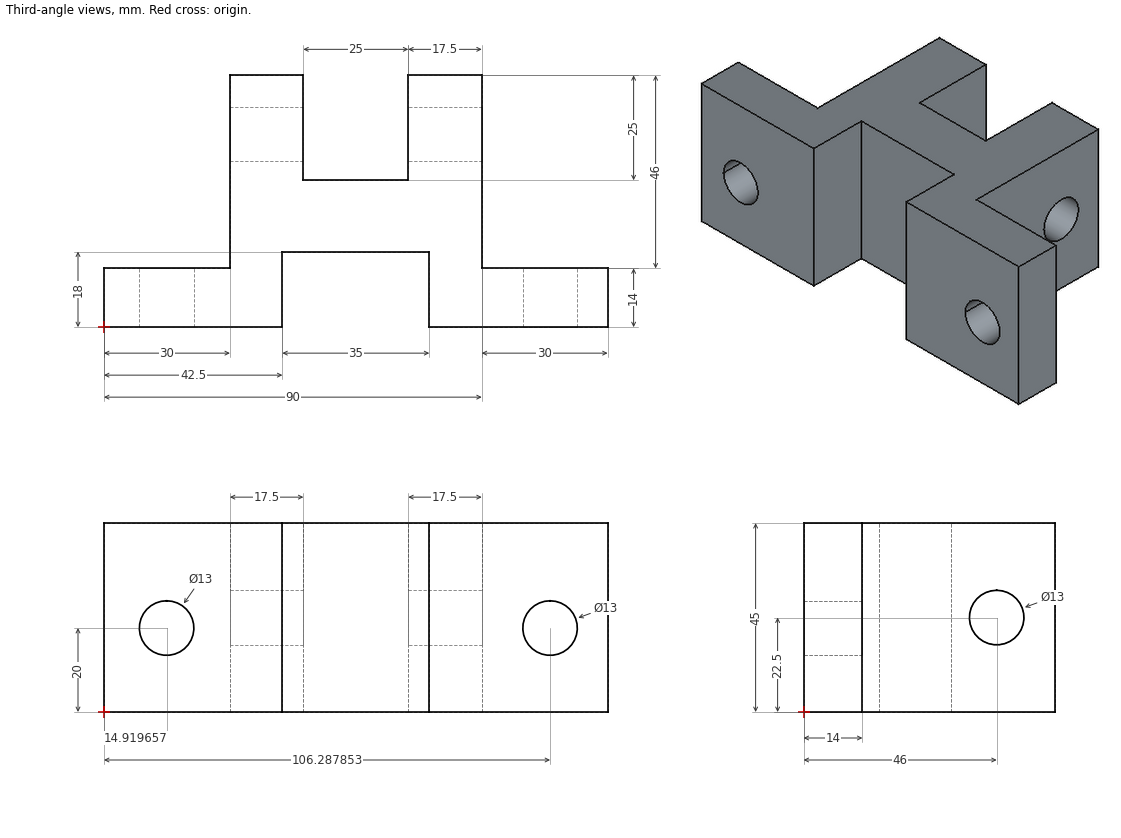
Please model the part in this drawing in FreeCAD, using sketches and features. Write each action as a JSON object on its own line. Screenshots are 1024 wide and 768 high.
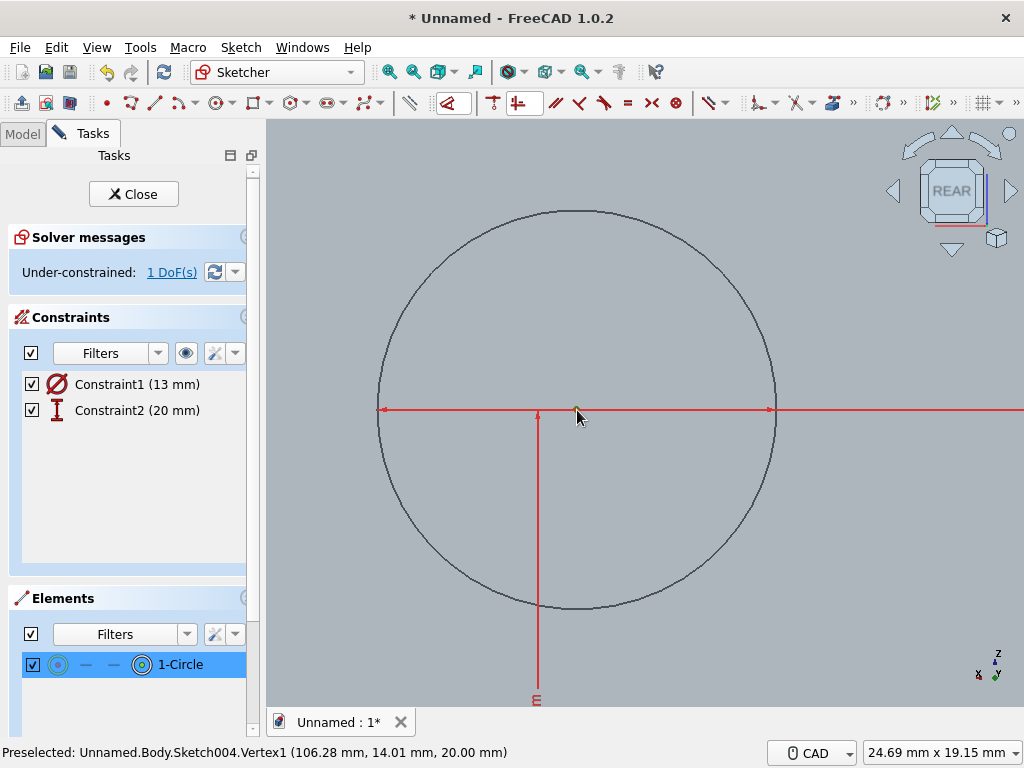
{"action": "key", "text": "l"}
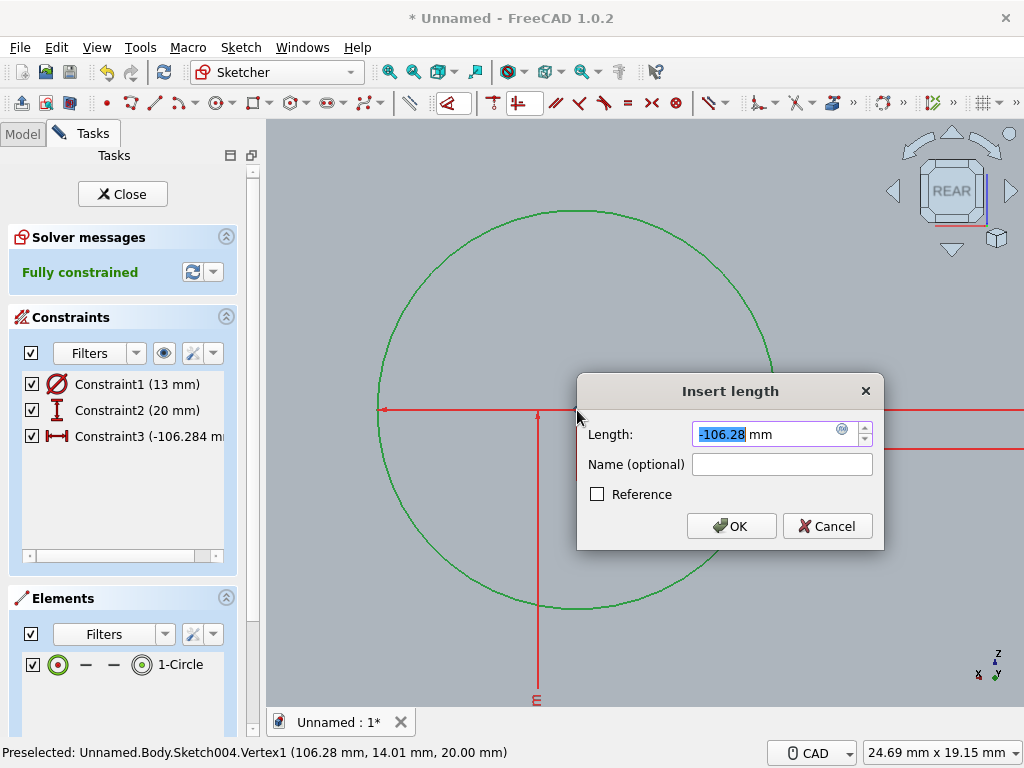
{"action": "type", "text": "-106.287853"}
{"action": "key", "text": "Return"}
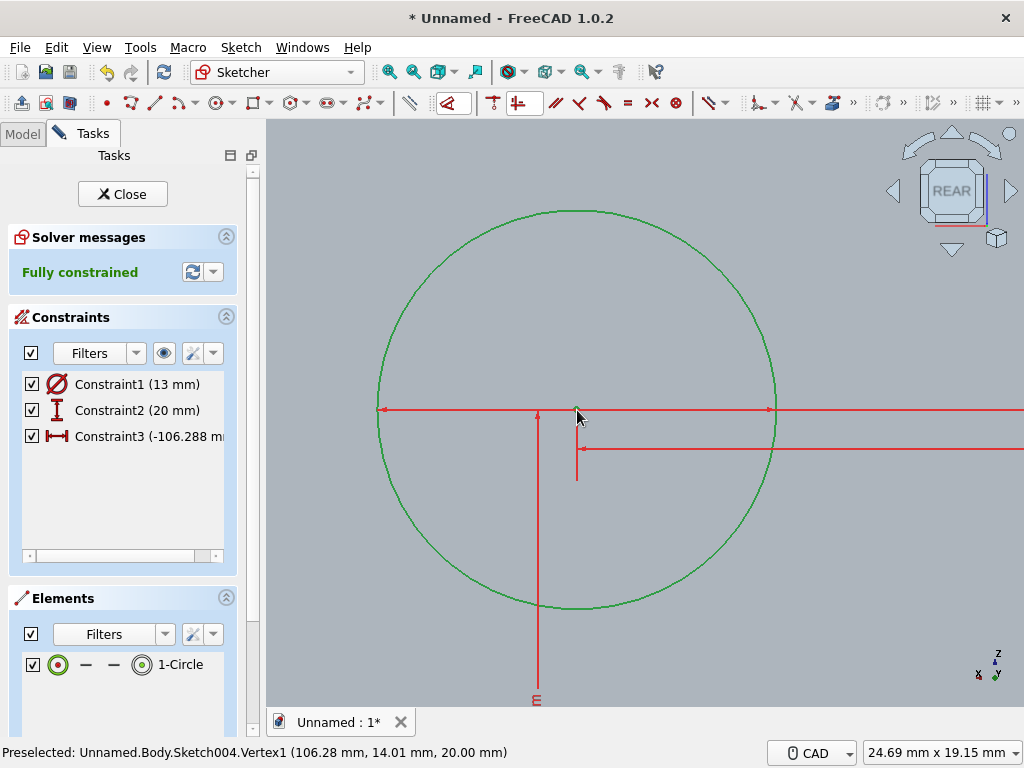
{"action": "left_click", "coordinate": [123, 194]}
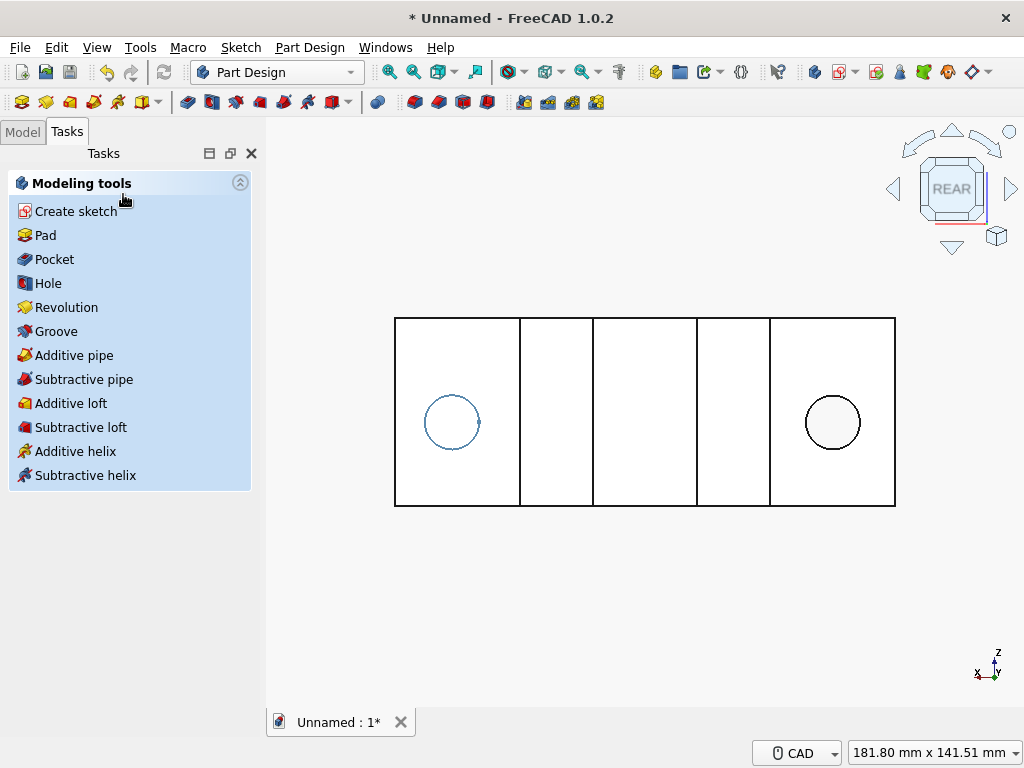
{"action": "left_click", "coordinate": [188, 102]}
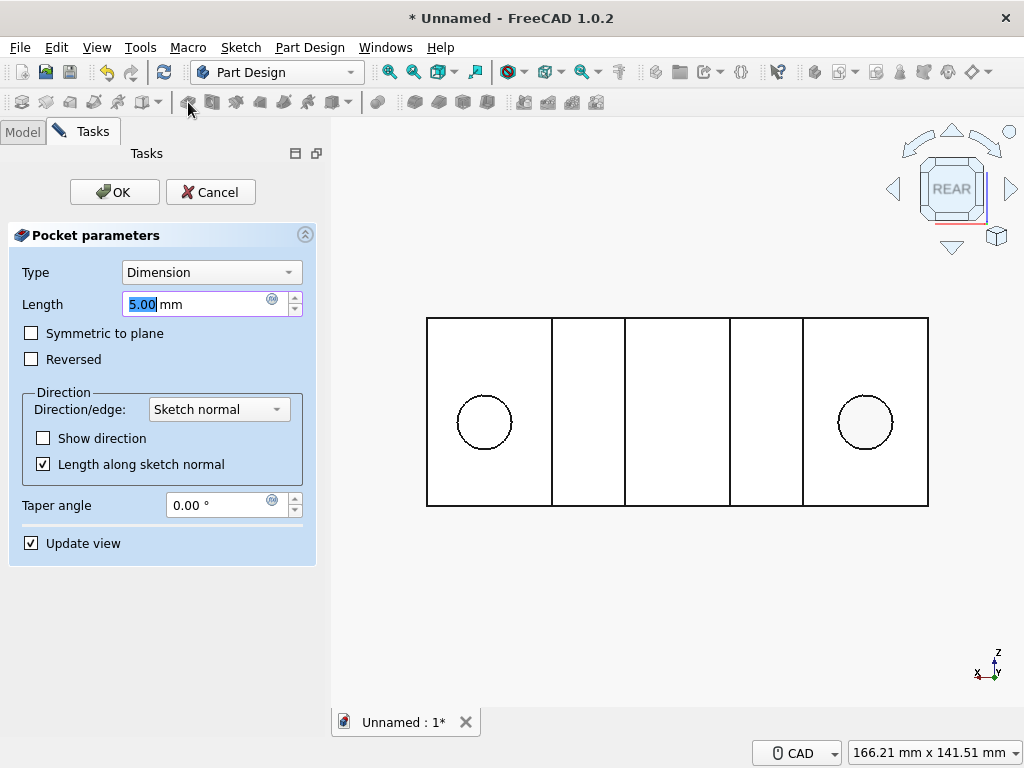
{"action": "type", "text": "14"}
{"action": "key", "text": "Tab"}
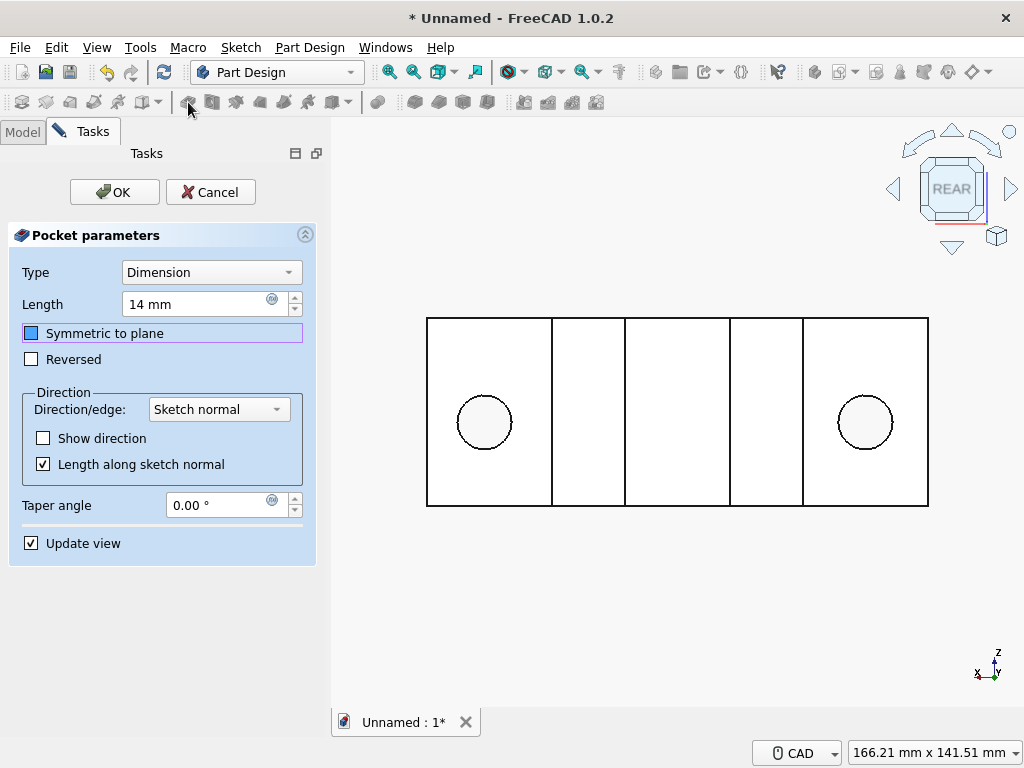
{"action": "left_click", "coordinate": [115, 192]}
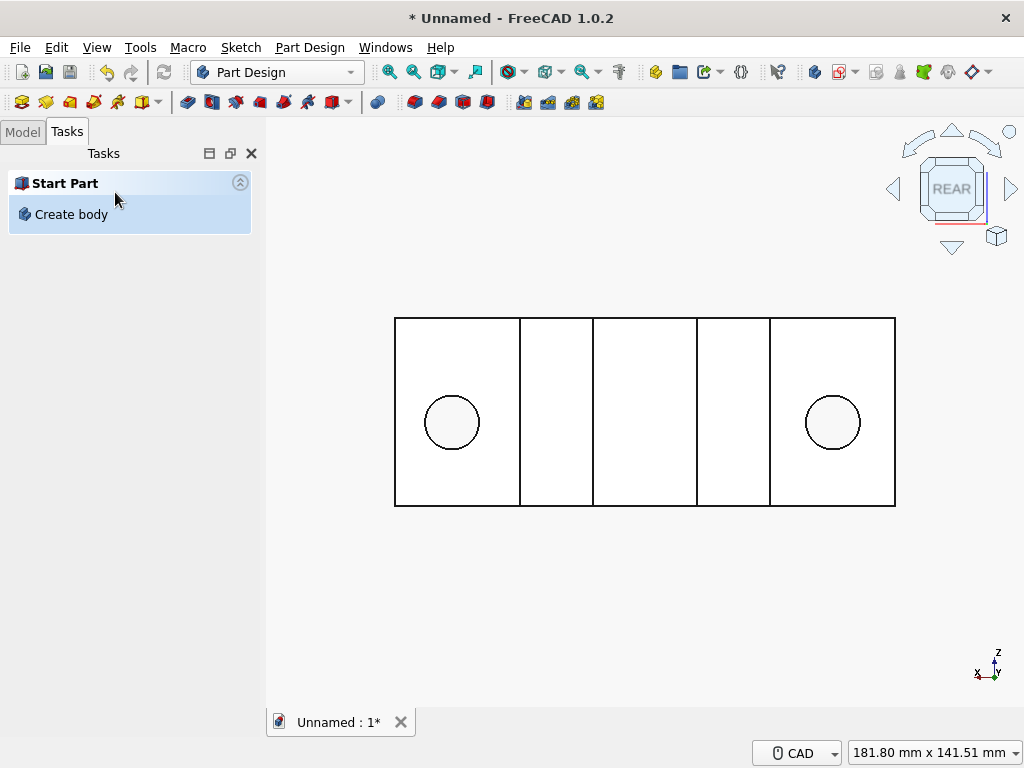
{"action": "key", "text": "0"}